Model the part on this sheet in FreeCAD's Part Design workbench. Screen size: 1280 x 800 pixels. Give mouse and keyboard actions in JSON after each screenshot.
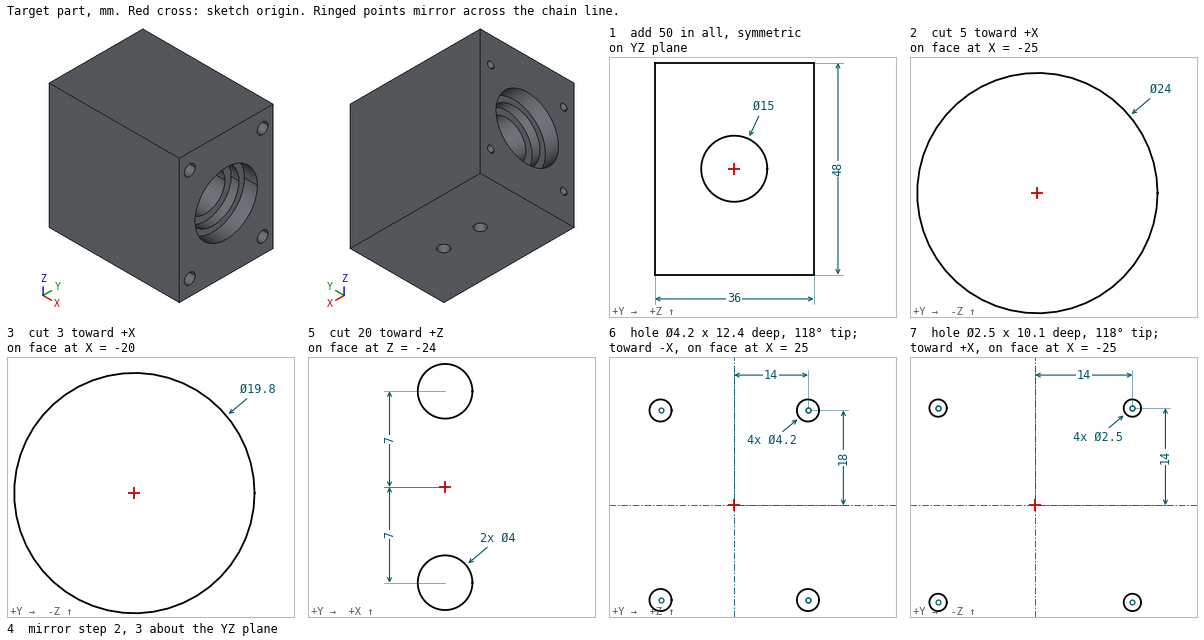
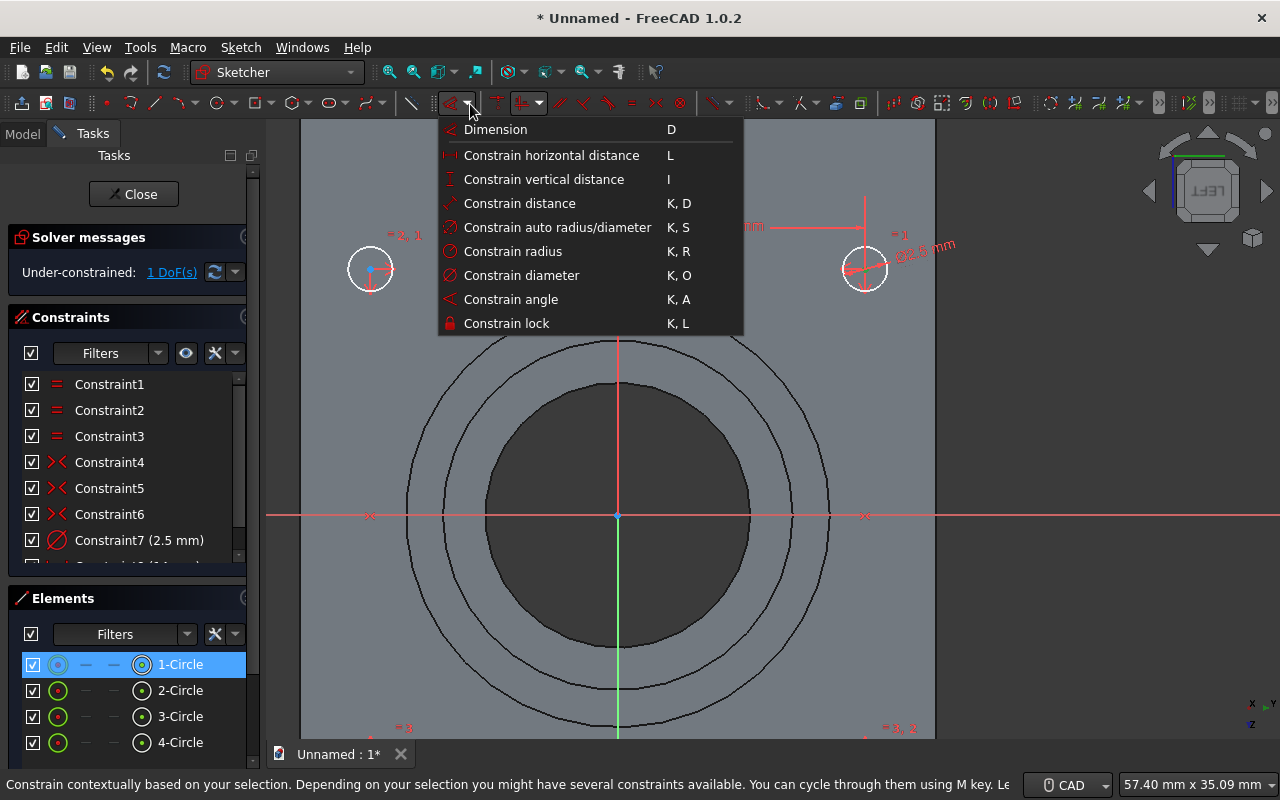
{"action": "left_click", "coordinate": [591, 179]}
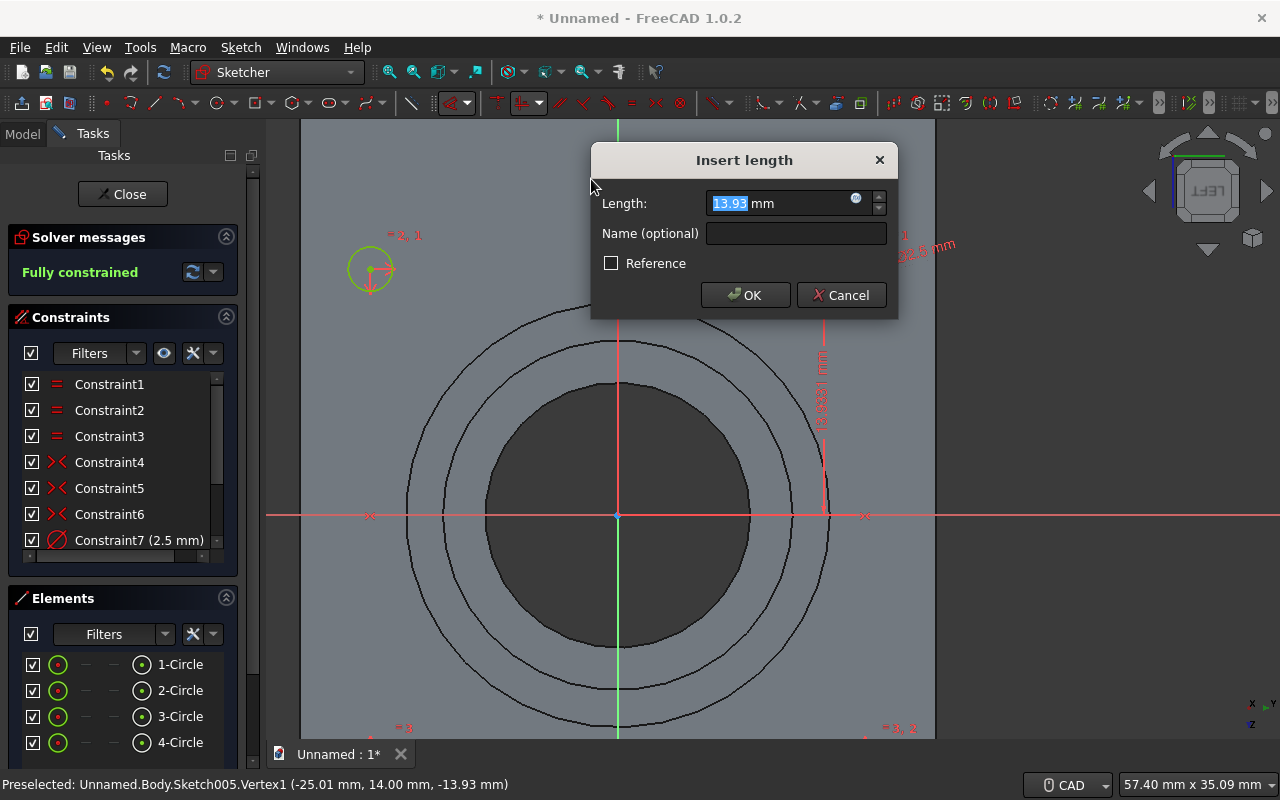
{"action": "type", "text": "14"}
{"action": "key", "text": "Return"}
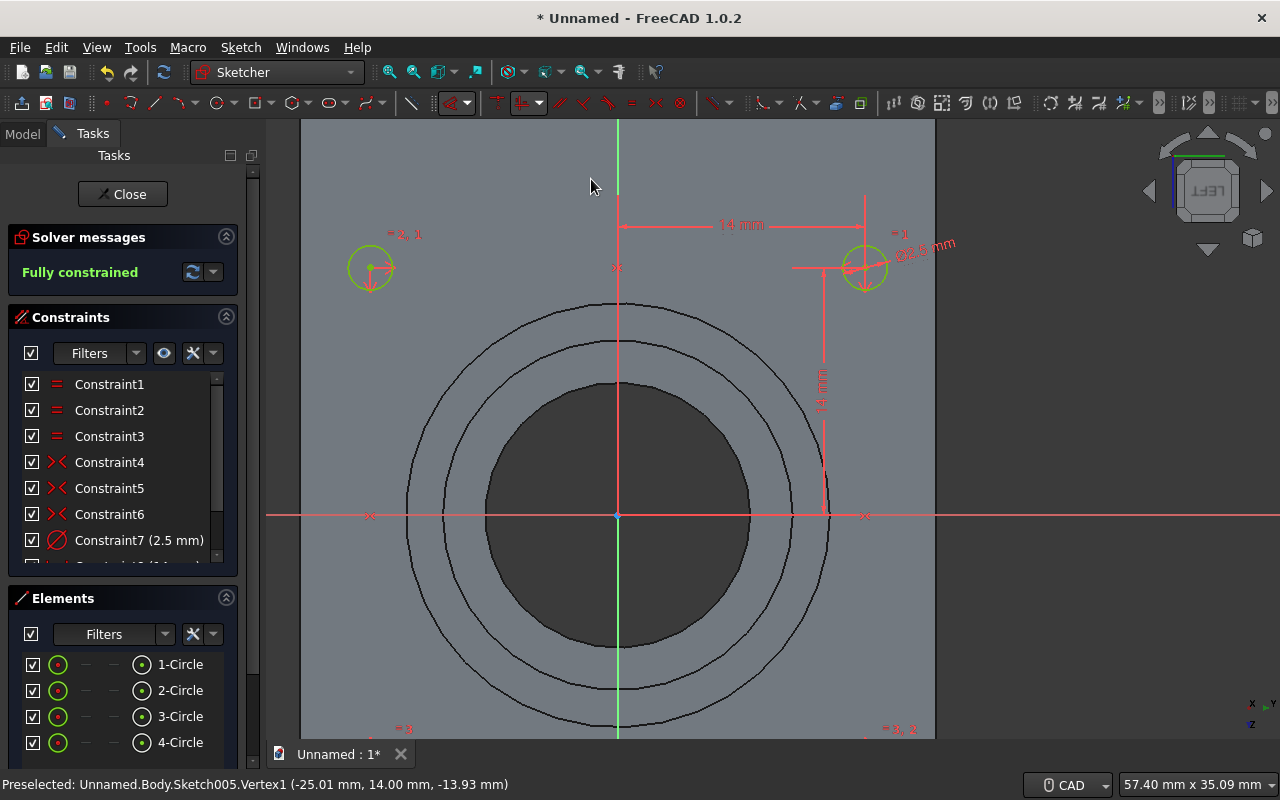
{"action": "left_click", "coordinate": [123, 194]}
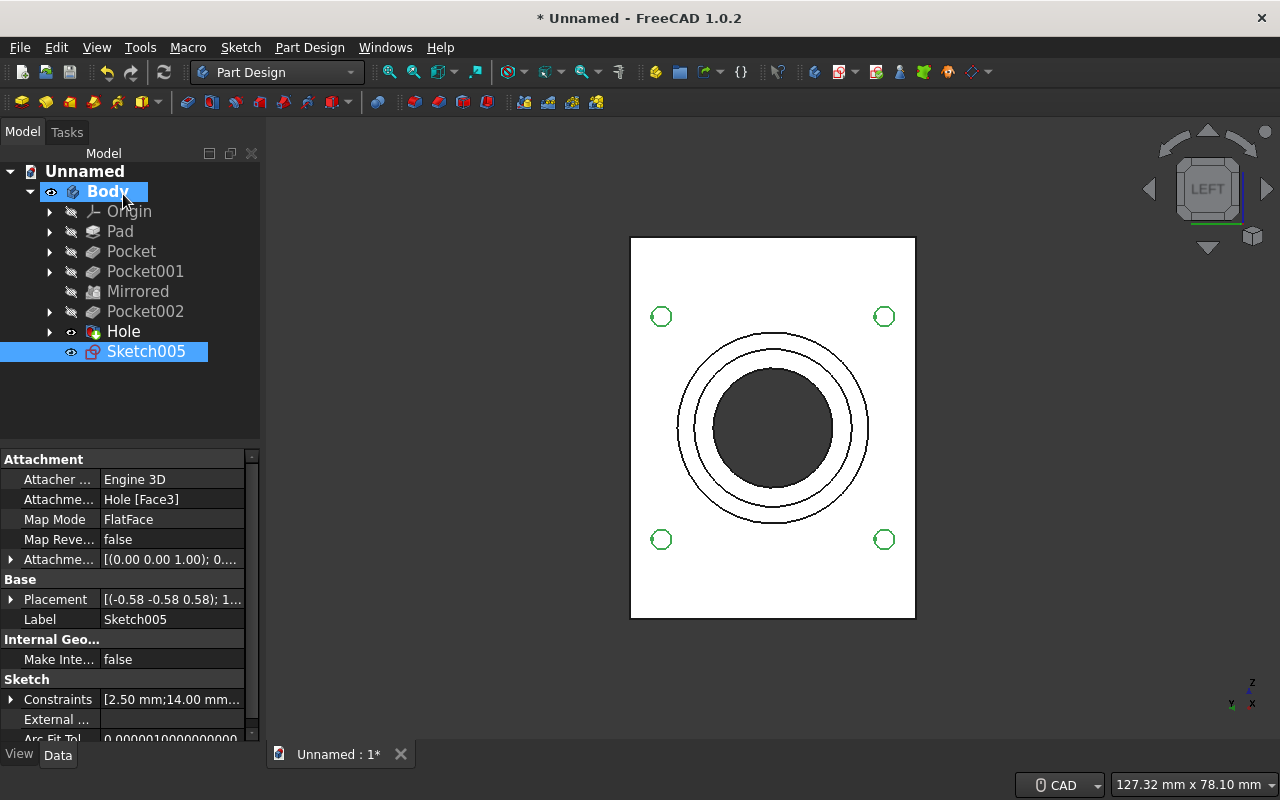
{"action": "left_click", "coordinate": [212, 102]}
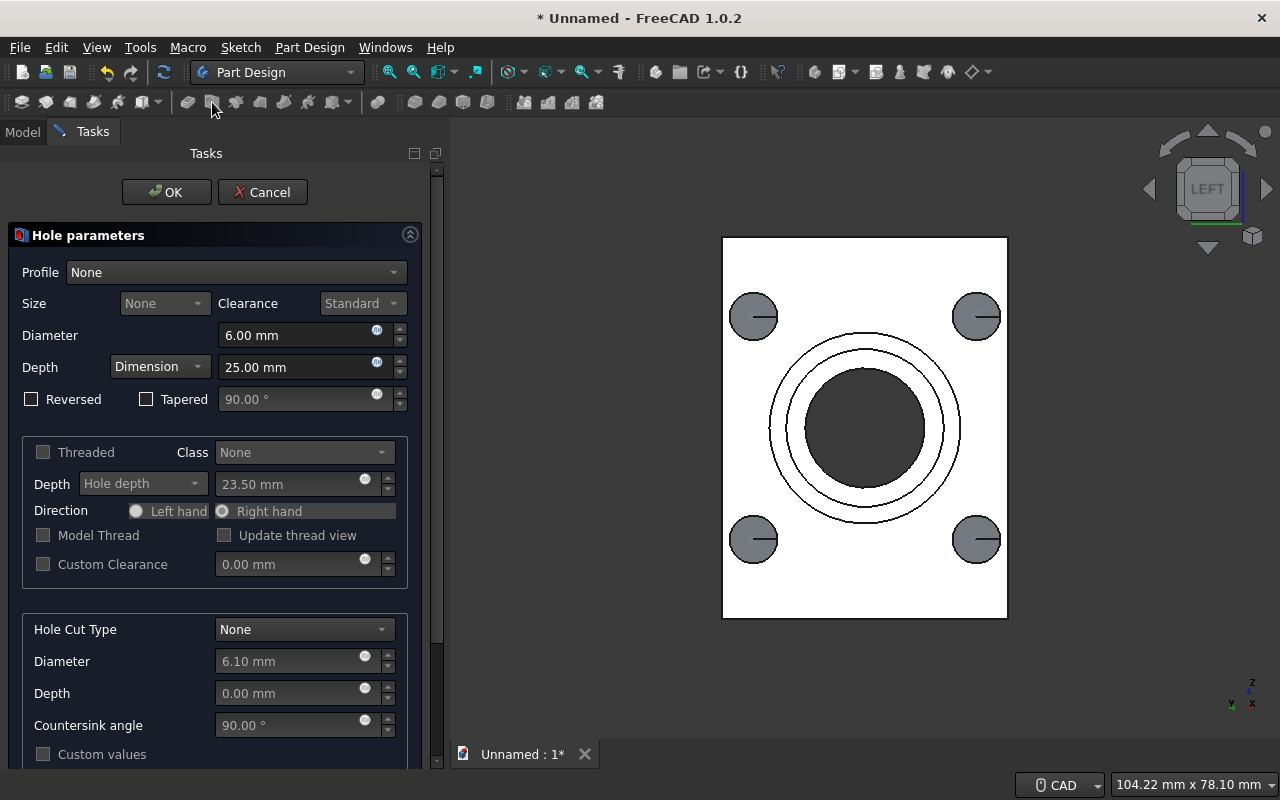
{"action": "triple_click", "coordinate": [305, 335]}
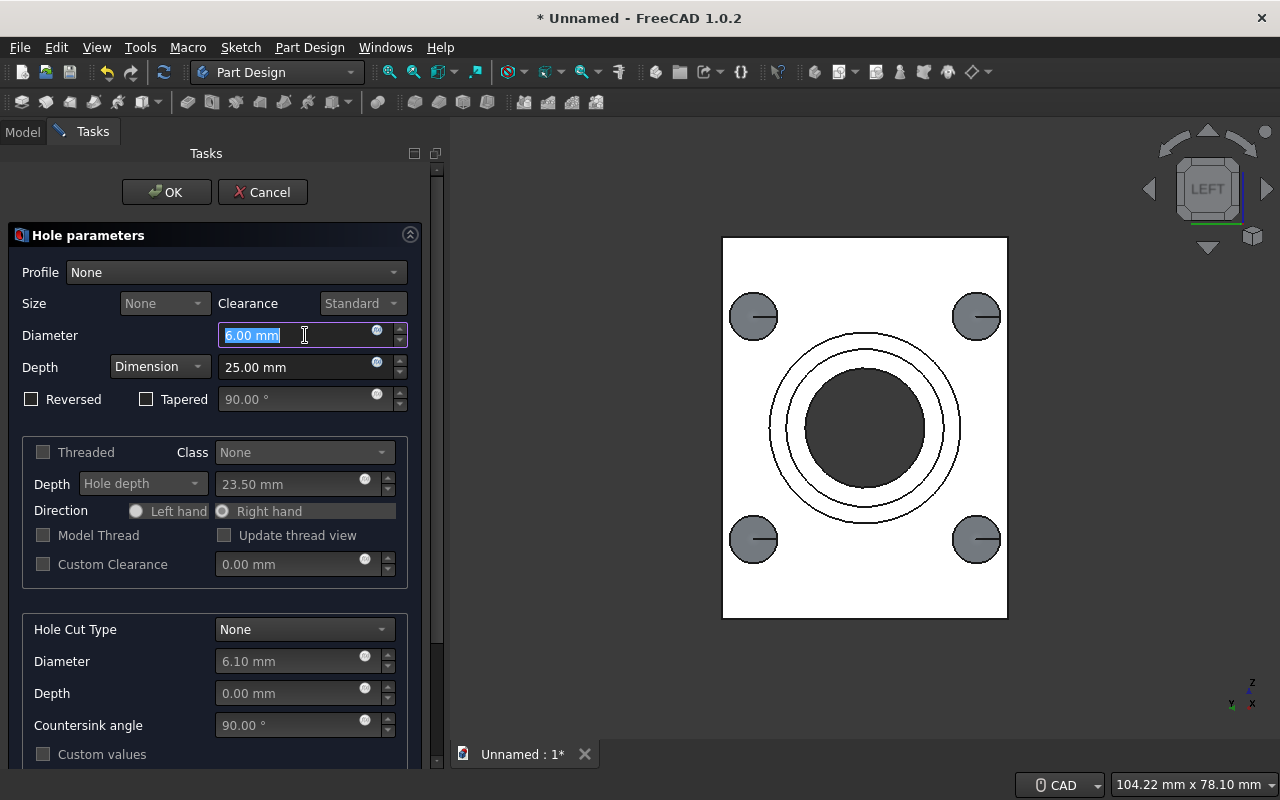
{"action": "type", "text": "2.5"}
{"action": "key", "text": "Tab"}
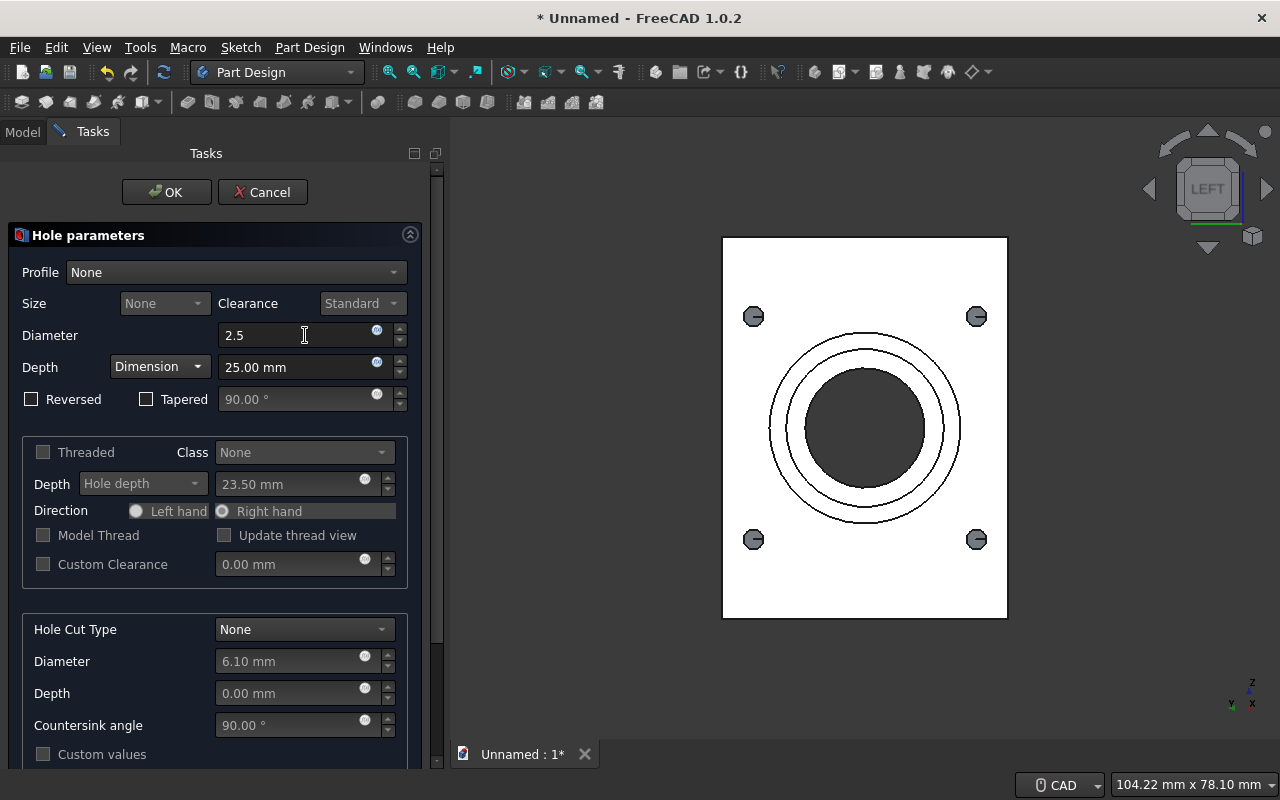
{"action": "triple_click", "coordinate": [305, 367]}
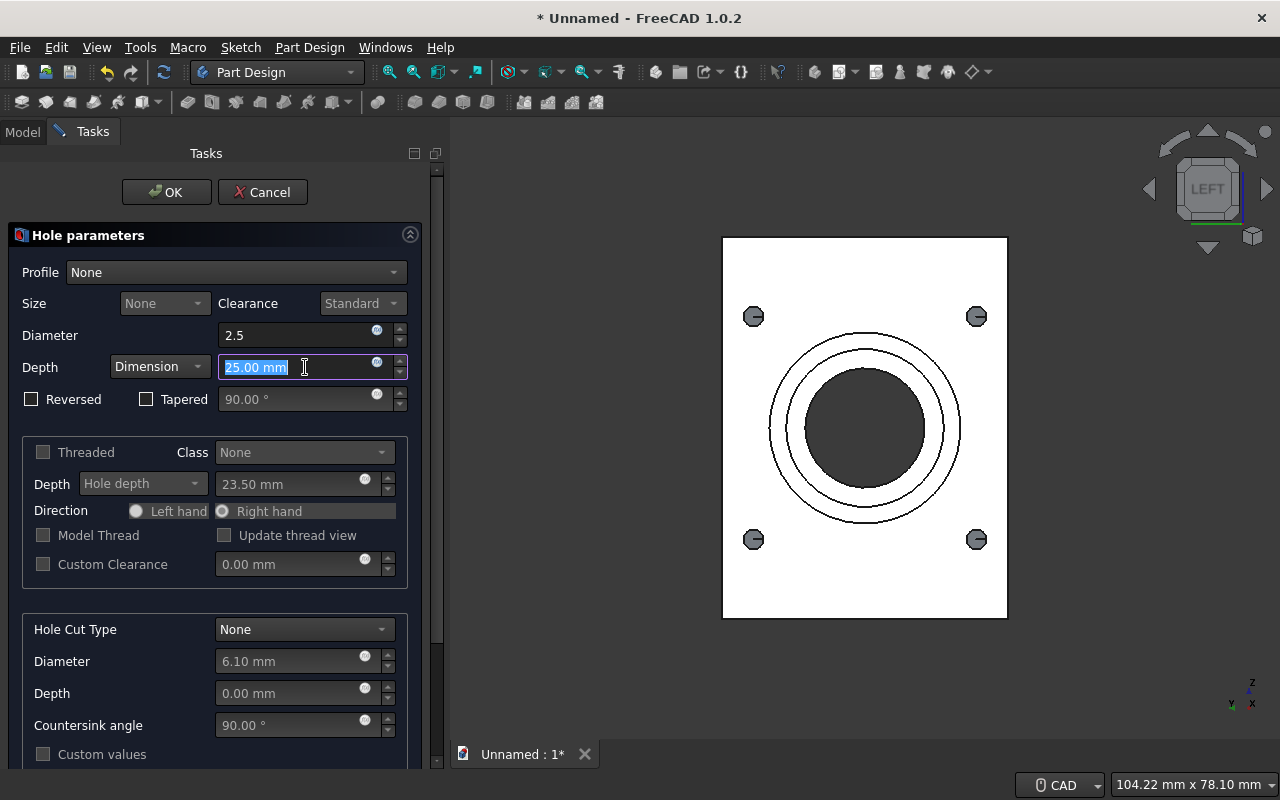
{"action": "type", "text": "10.1"}
{"action": "key", "text": "Tab"}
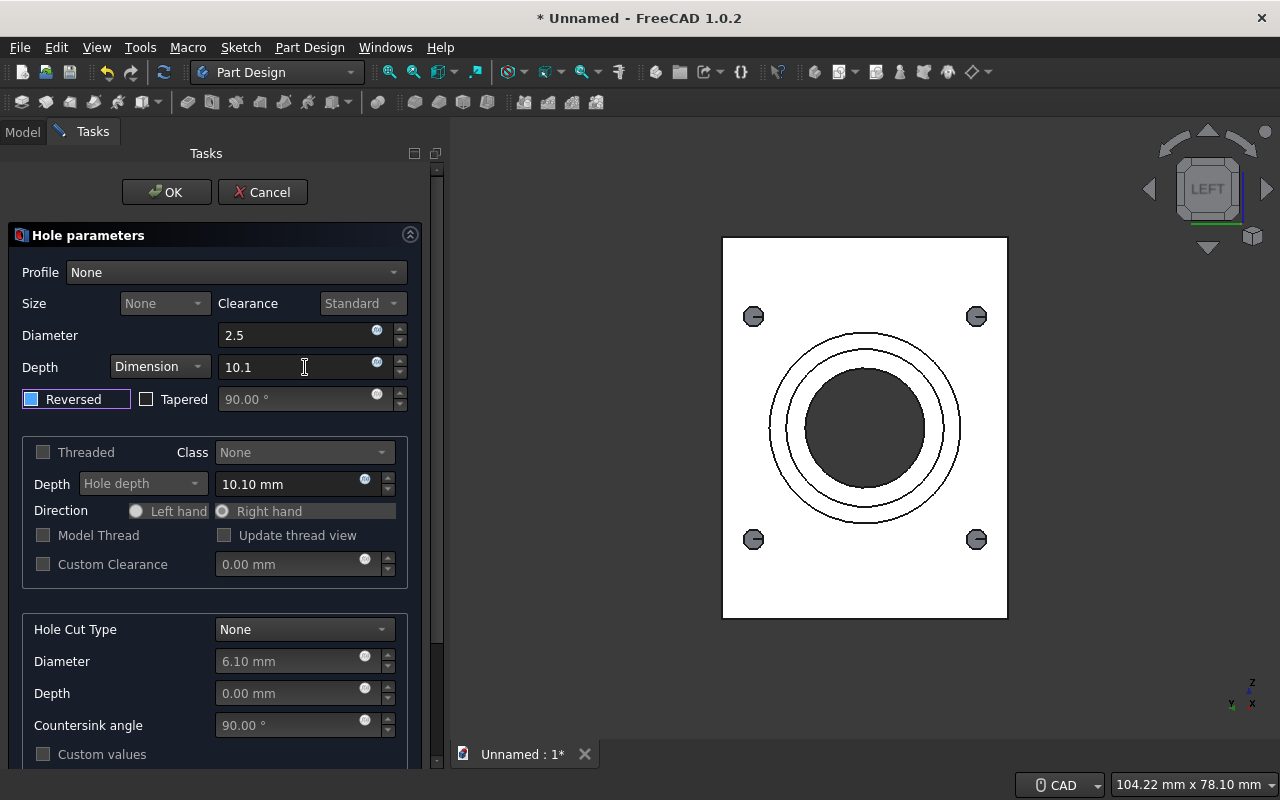
{"action": "left_click", "coordinate": [167, 192]}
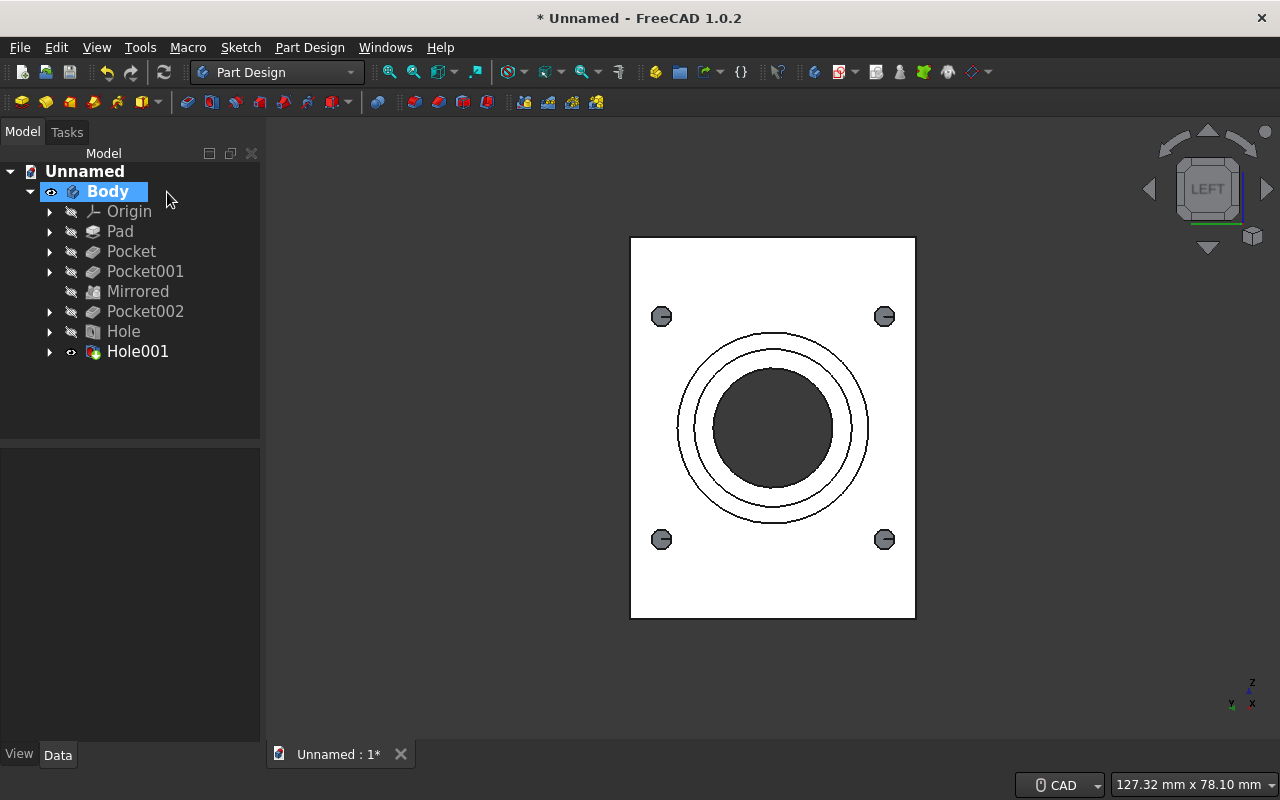
{"action": "key", "text": "0"}